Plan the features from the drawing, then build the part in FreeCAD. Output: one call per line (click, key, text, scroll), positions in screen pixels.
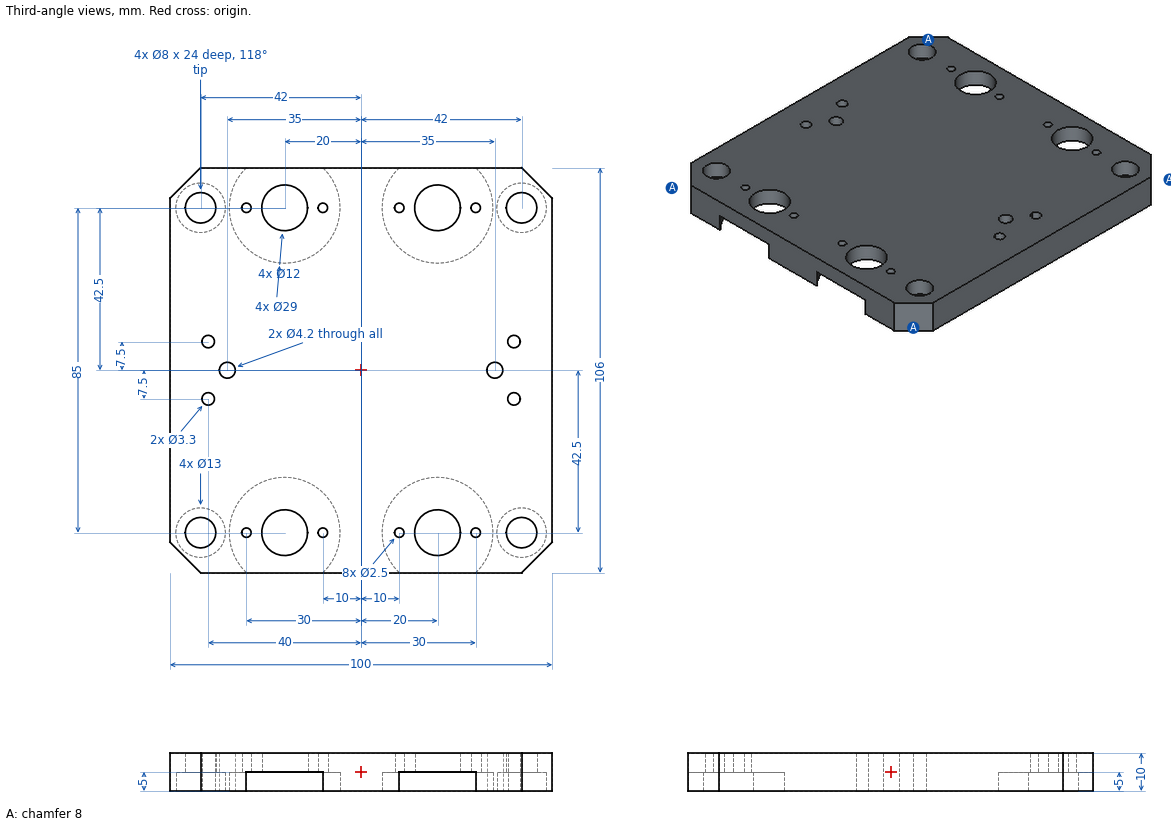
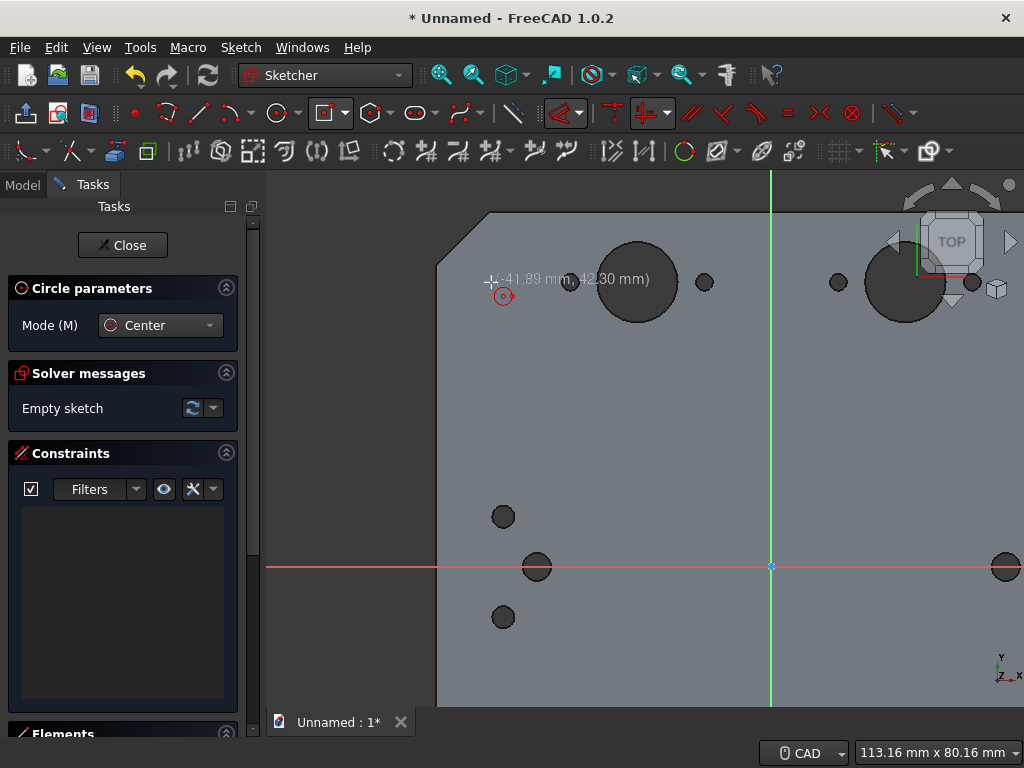
click(490, 282)
move(509, 263)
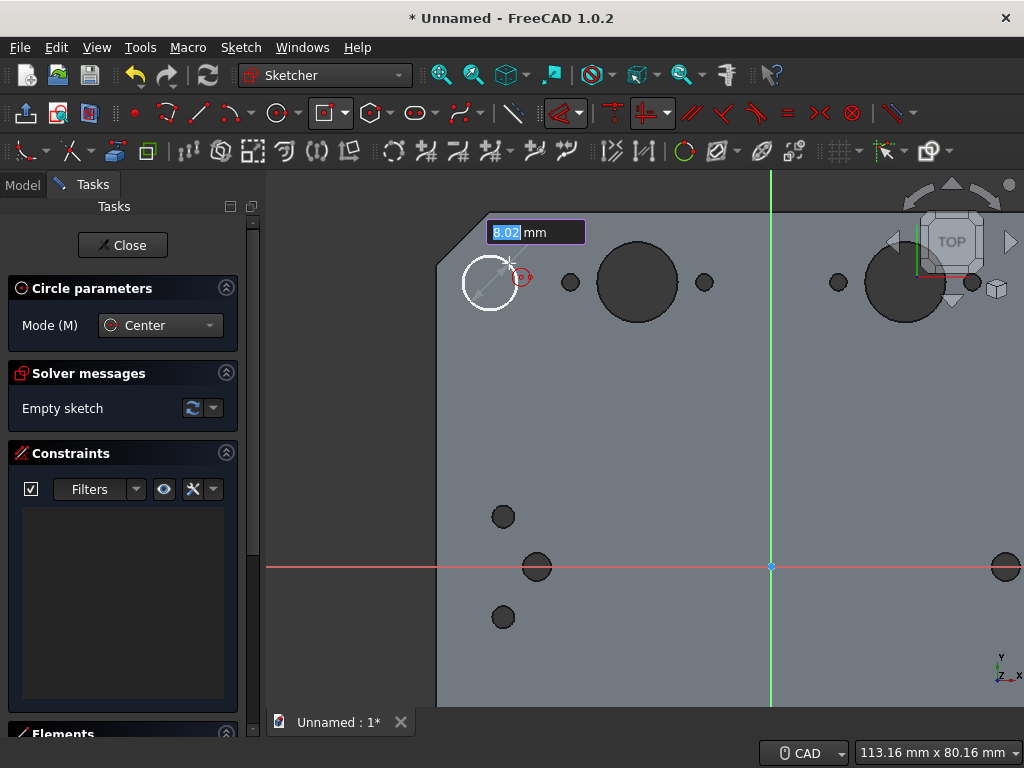
text(8)
key(Return)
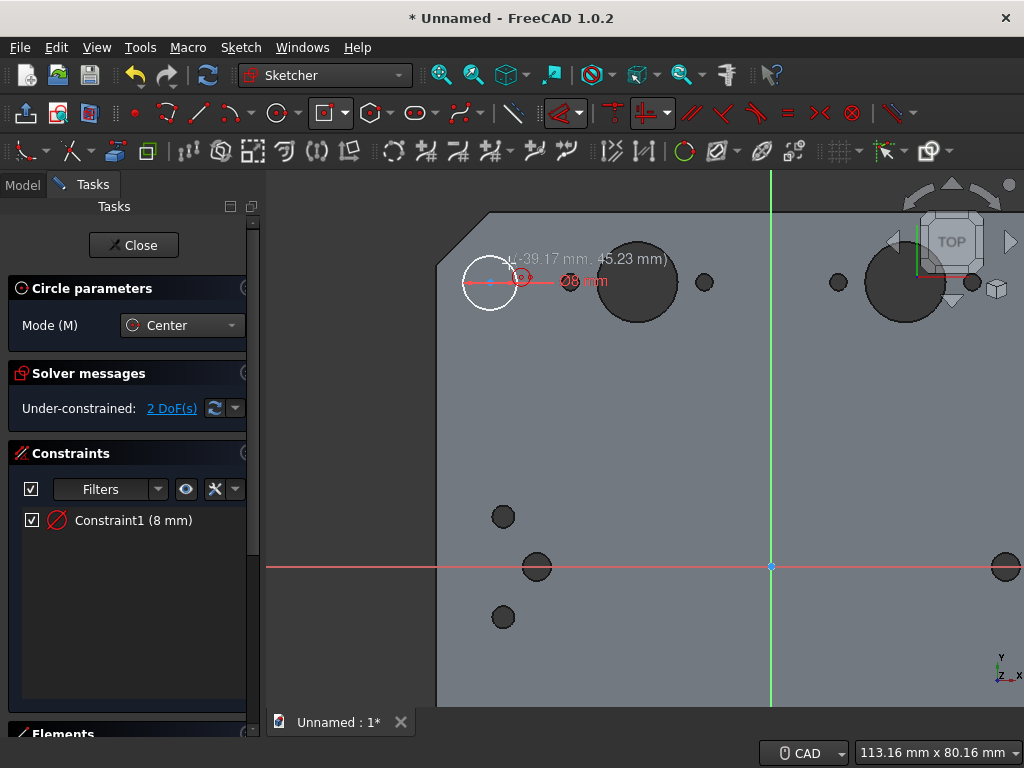
scroll(339, 282, down, 3)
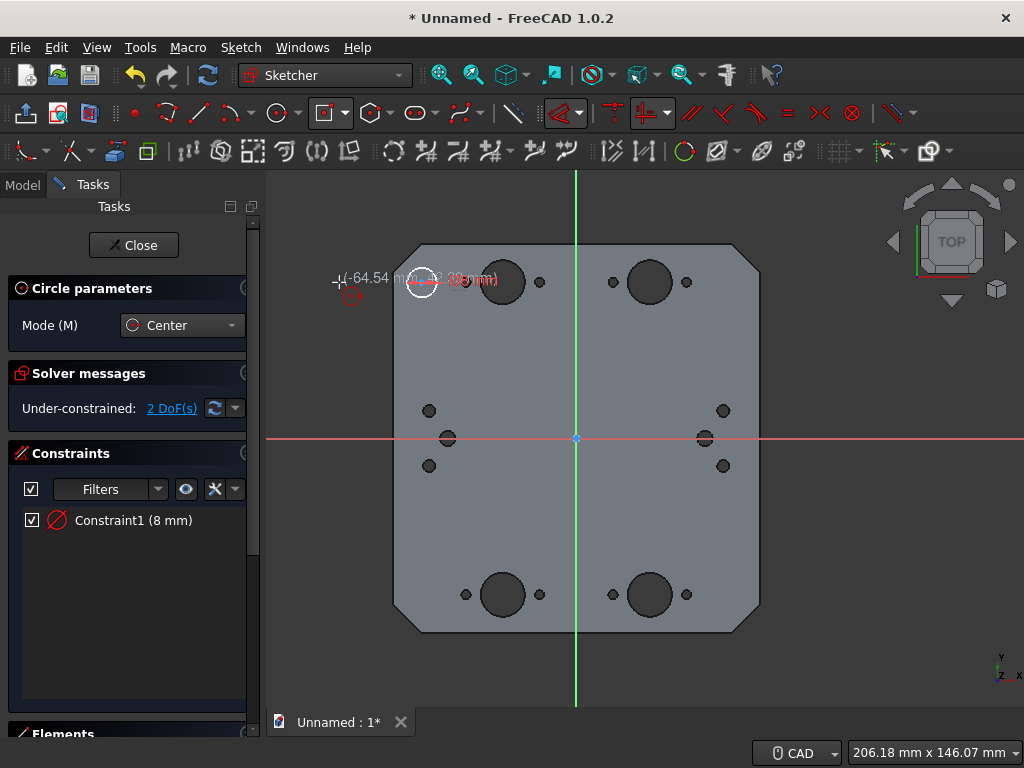
scroll(731, 282, up, 3)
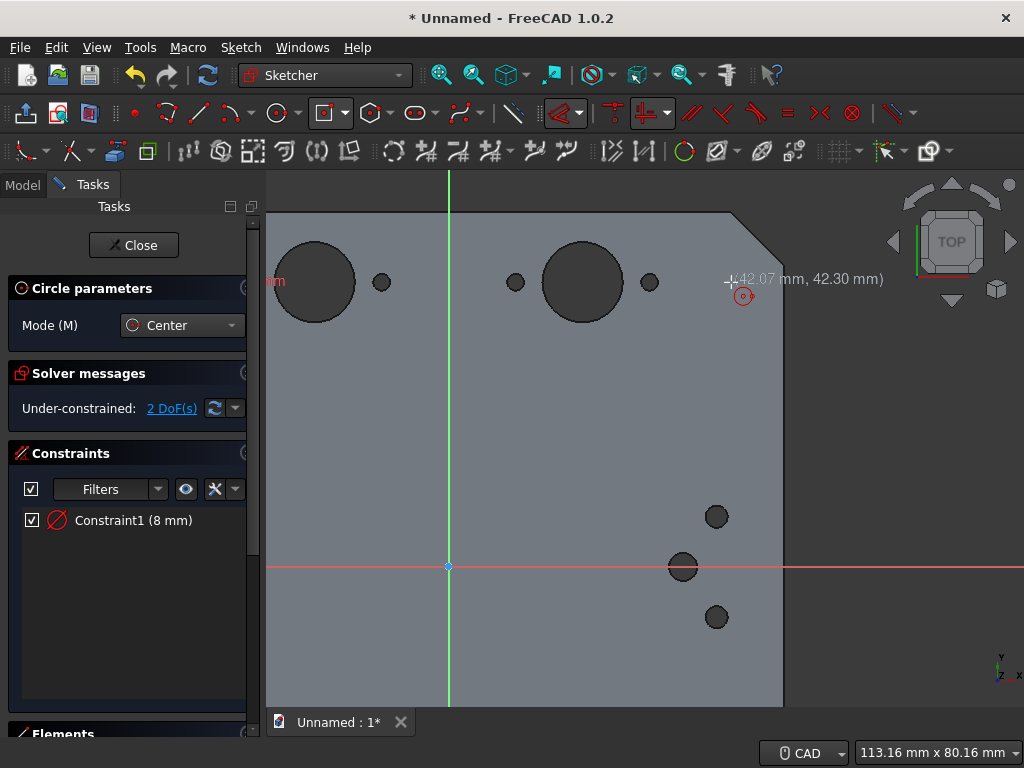
click(730, 282)
move(749, 263)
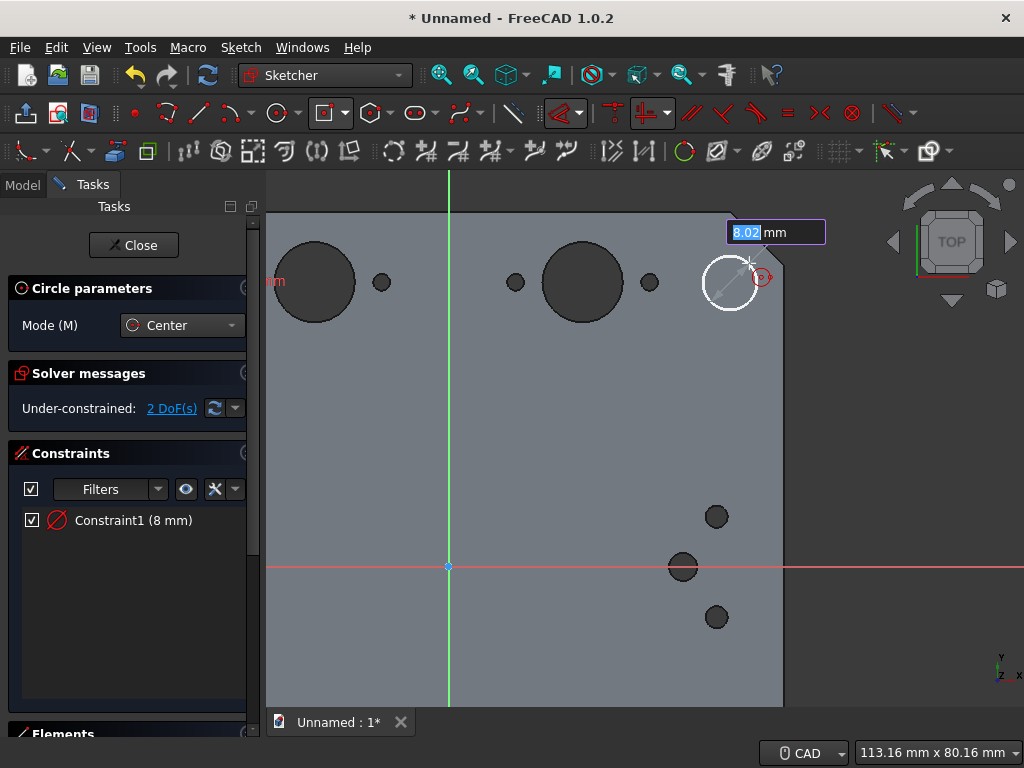
text(8)
key(Return)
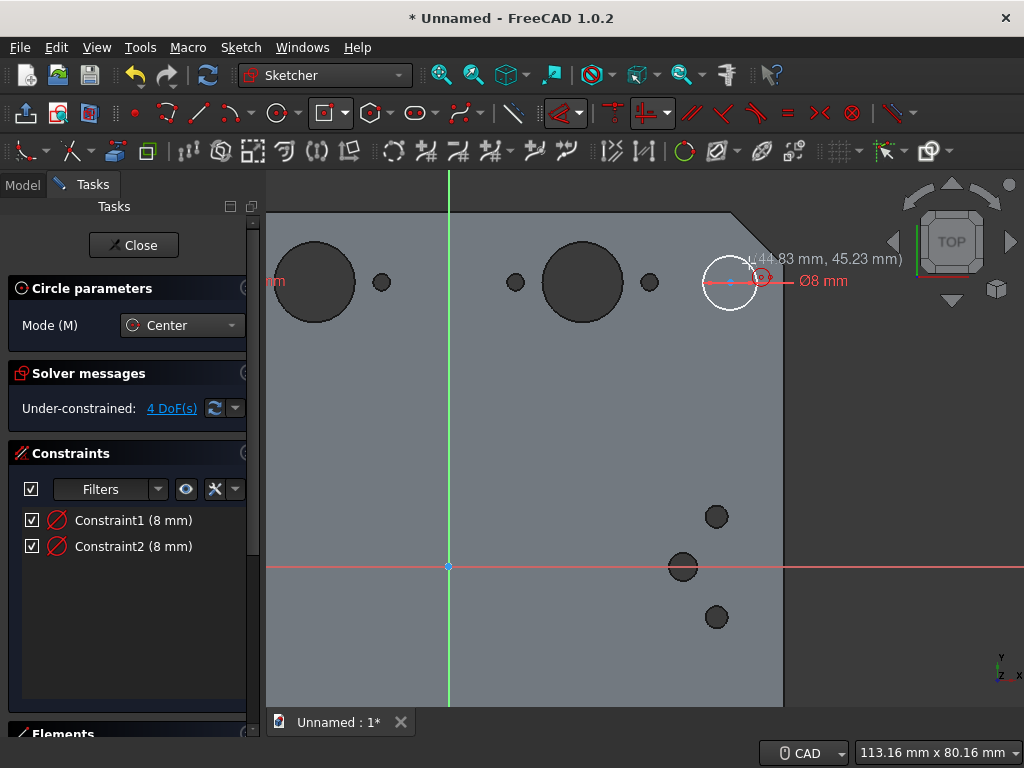
scroll(732, 282, down, 3)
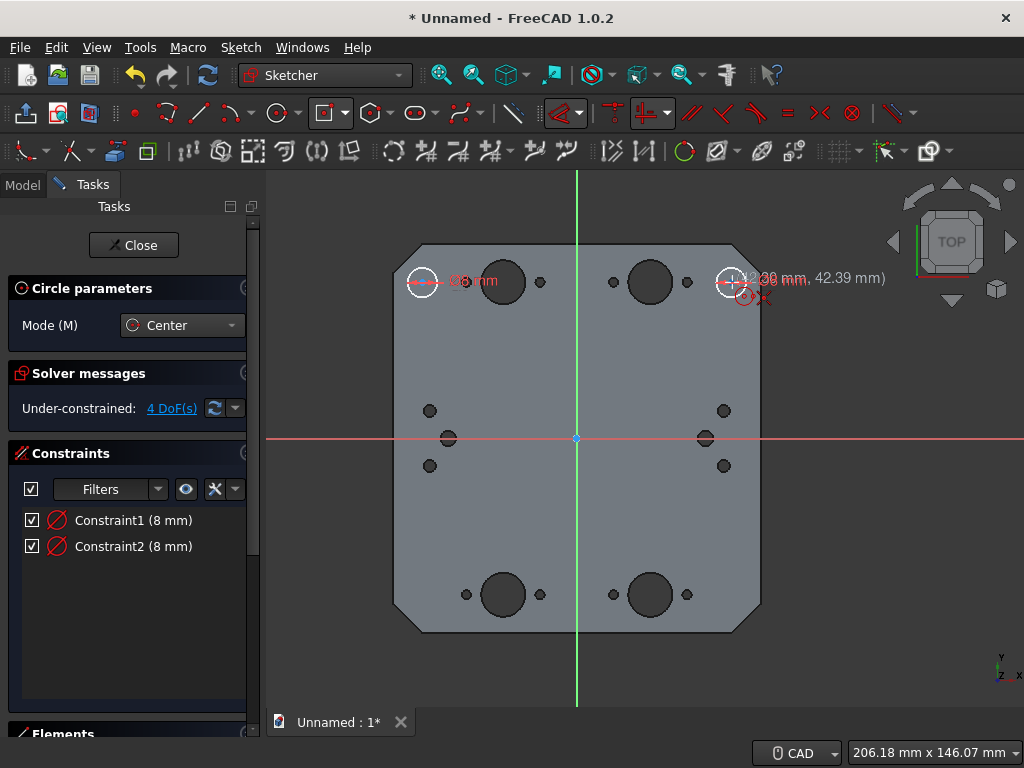
scroll(731, 595, up, 3)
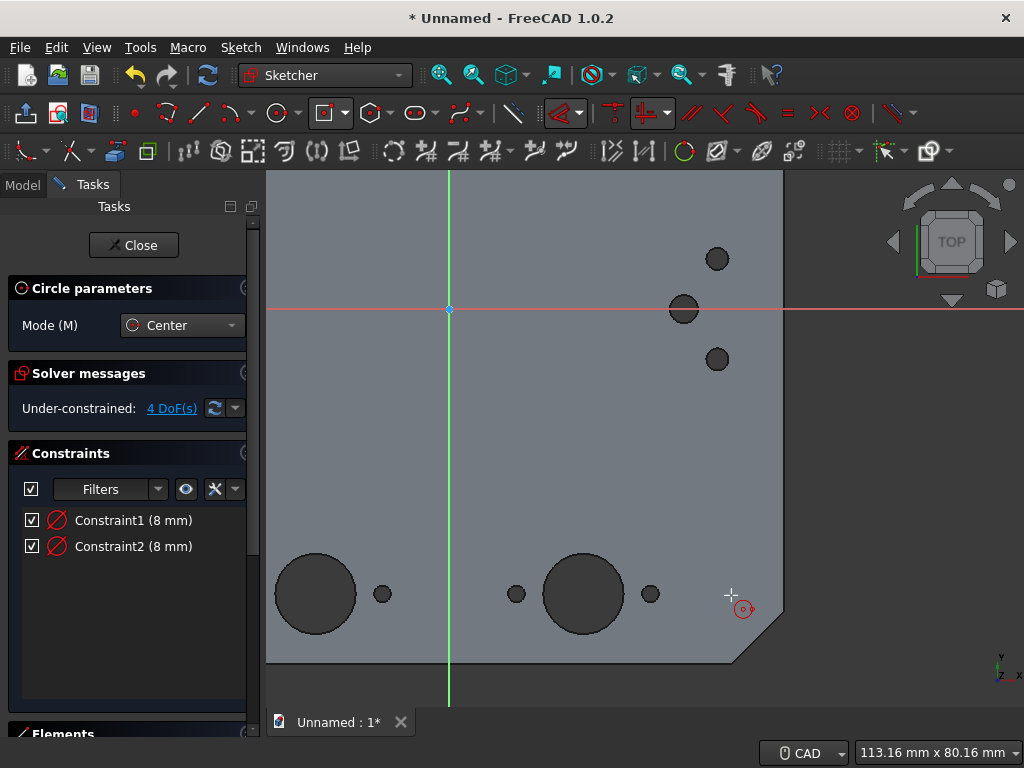
click(731, 594)
move(750, 575)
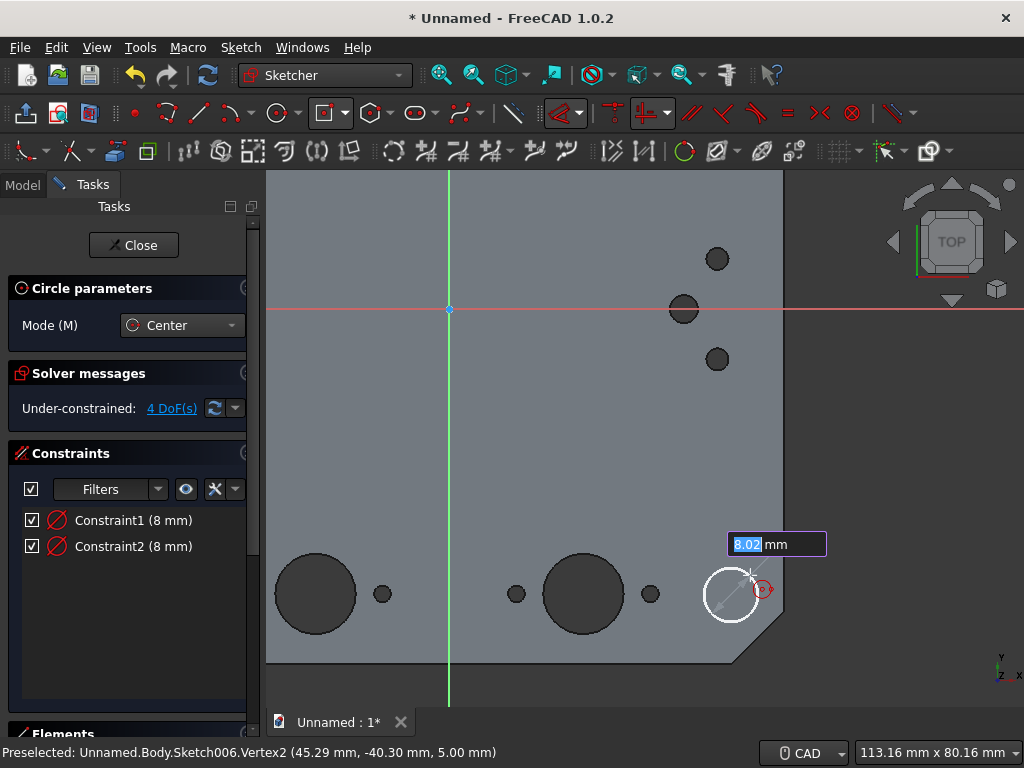
text(8)
key(Return)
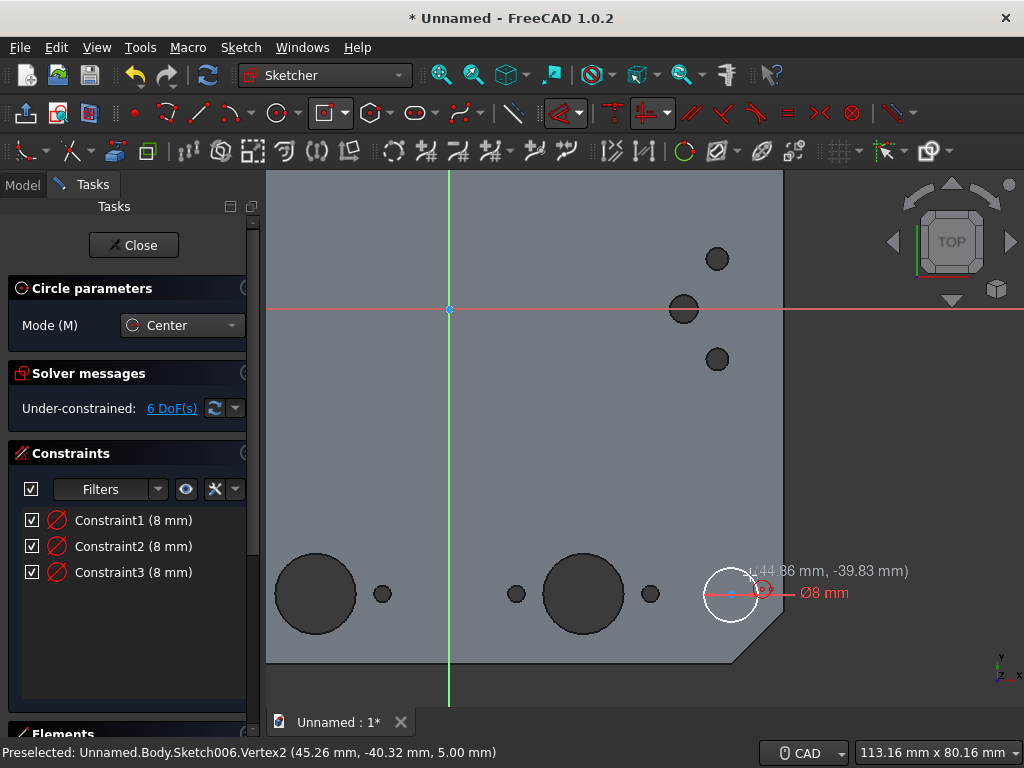
scroll(731, 596, down, 3)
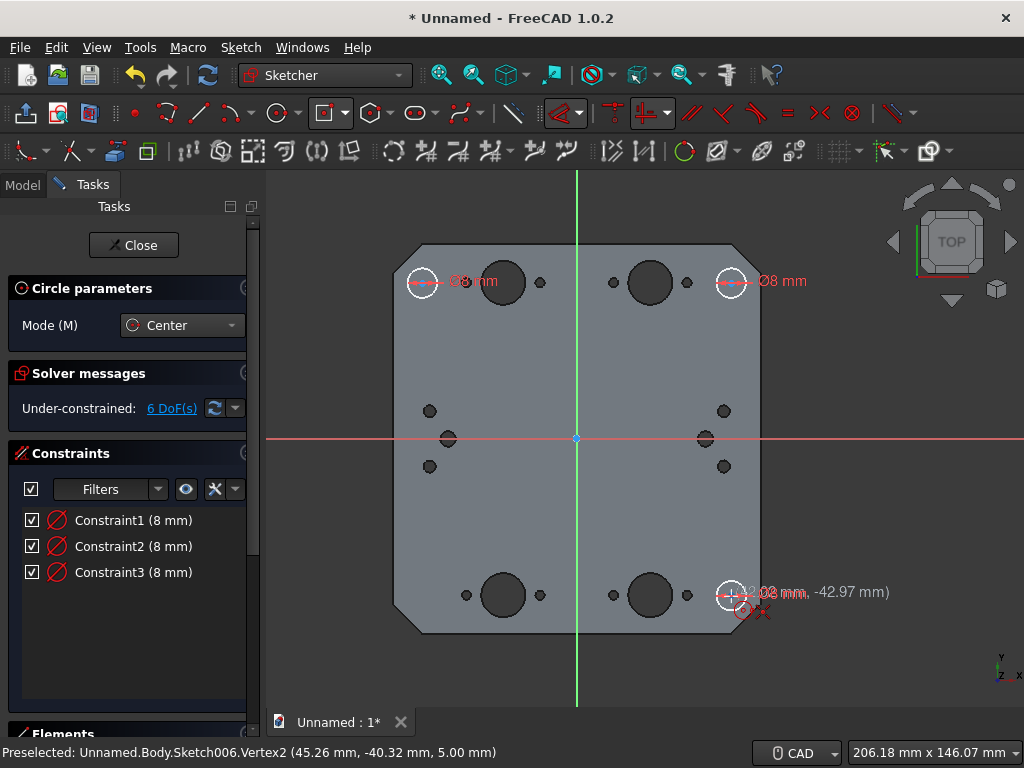
scroll(422, 595, up, 3)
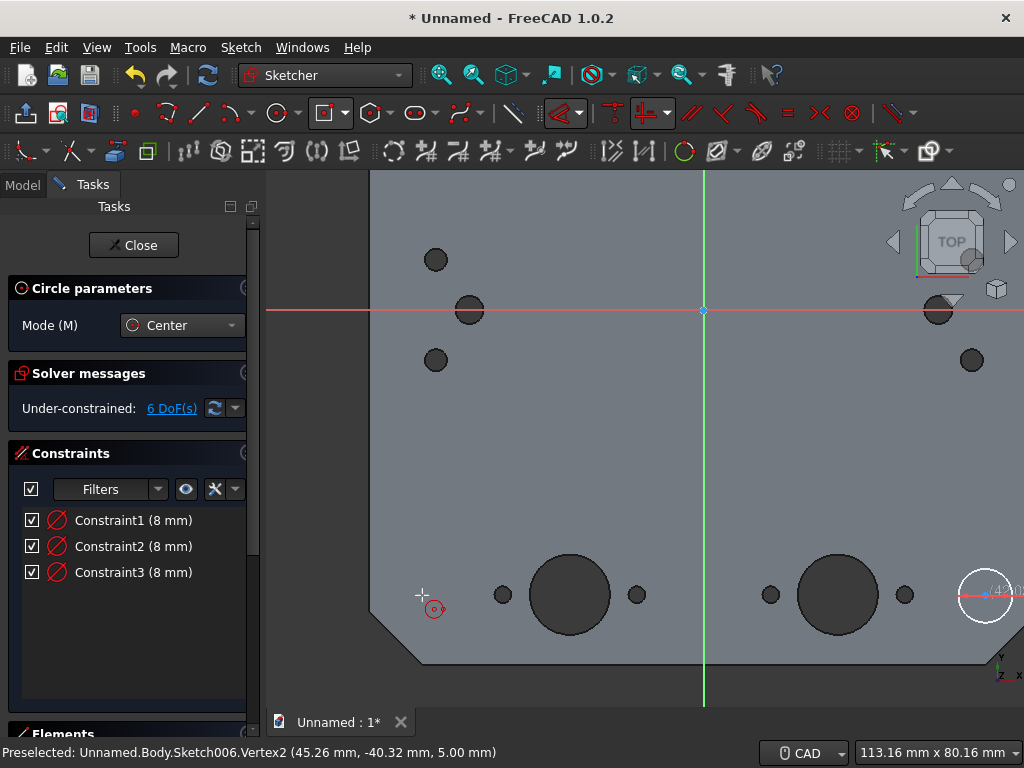
click(423, 595)
move(441, 576)